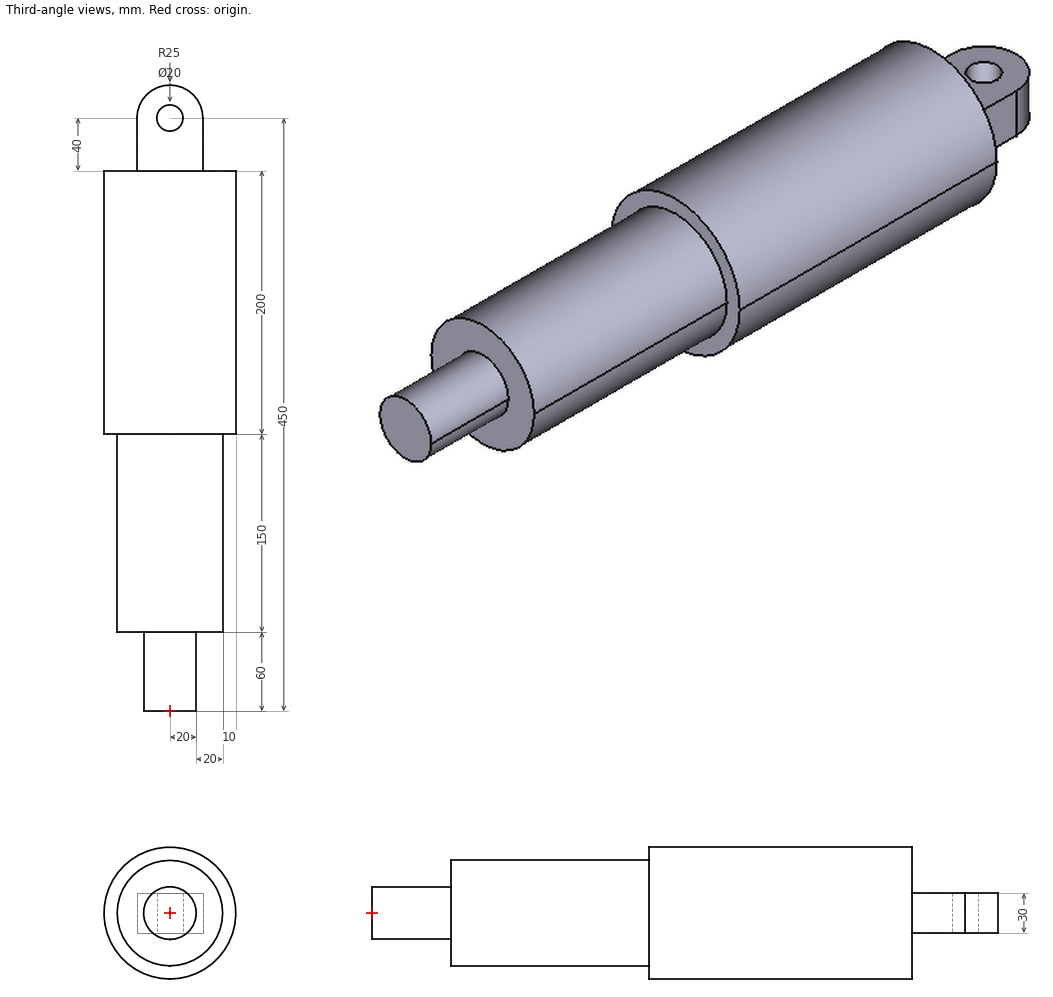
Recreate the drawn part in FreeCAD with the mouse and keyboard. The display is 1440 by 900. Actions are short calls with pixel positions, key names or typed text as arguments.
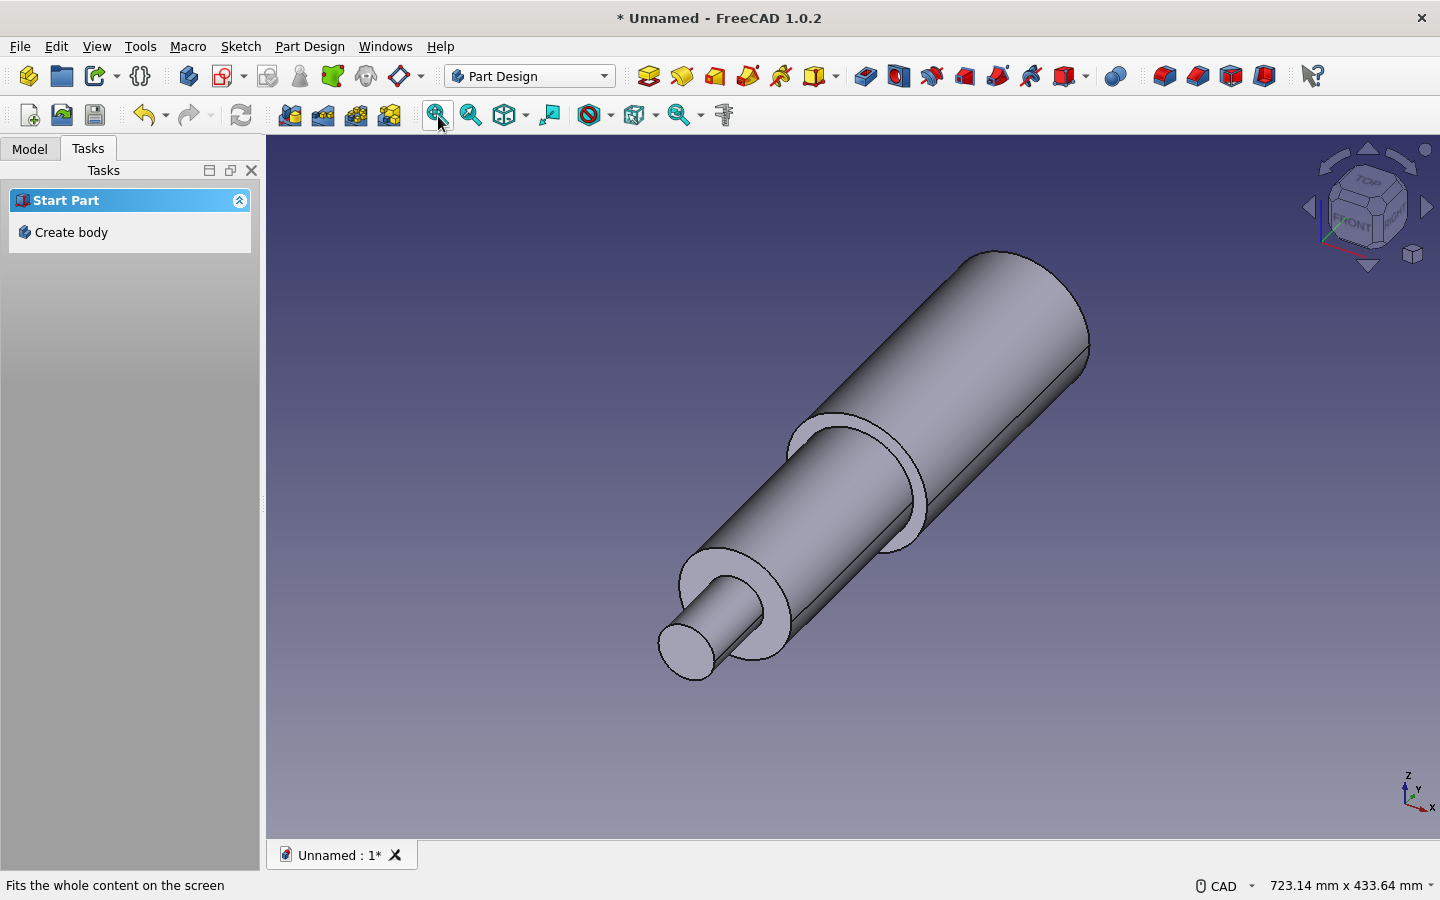
click(222, 76)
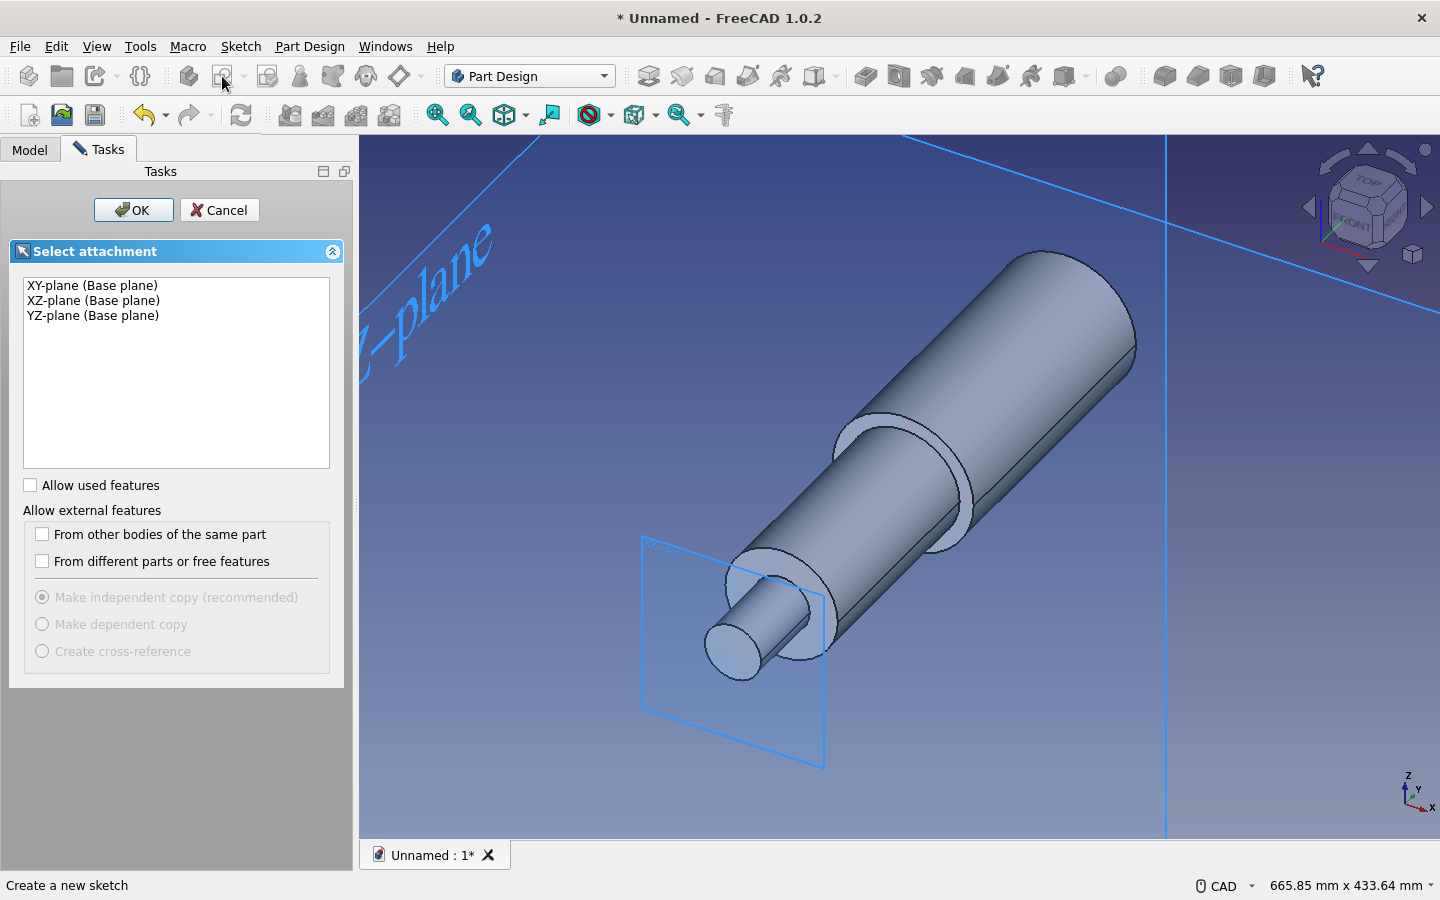
click(84, 286)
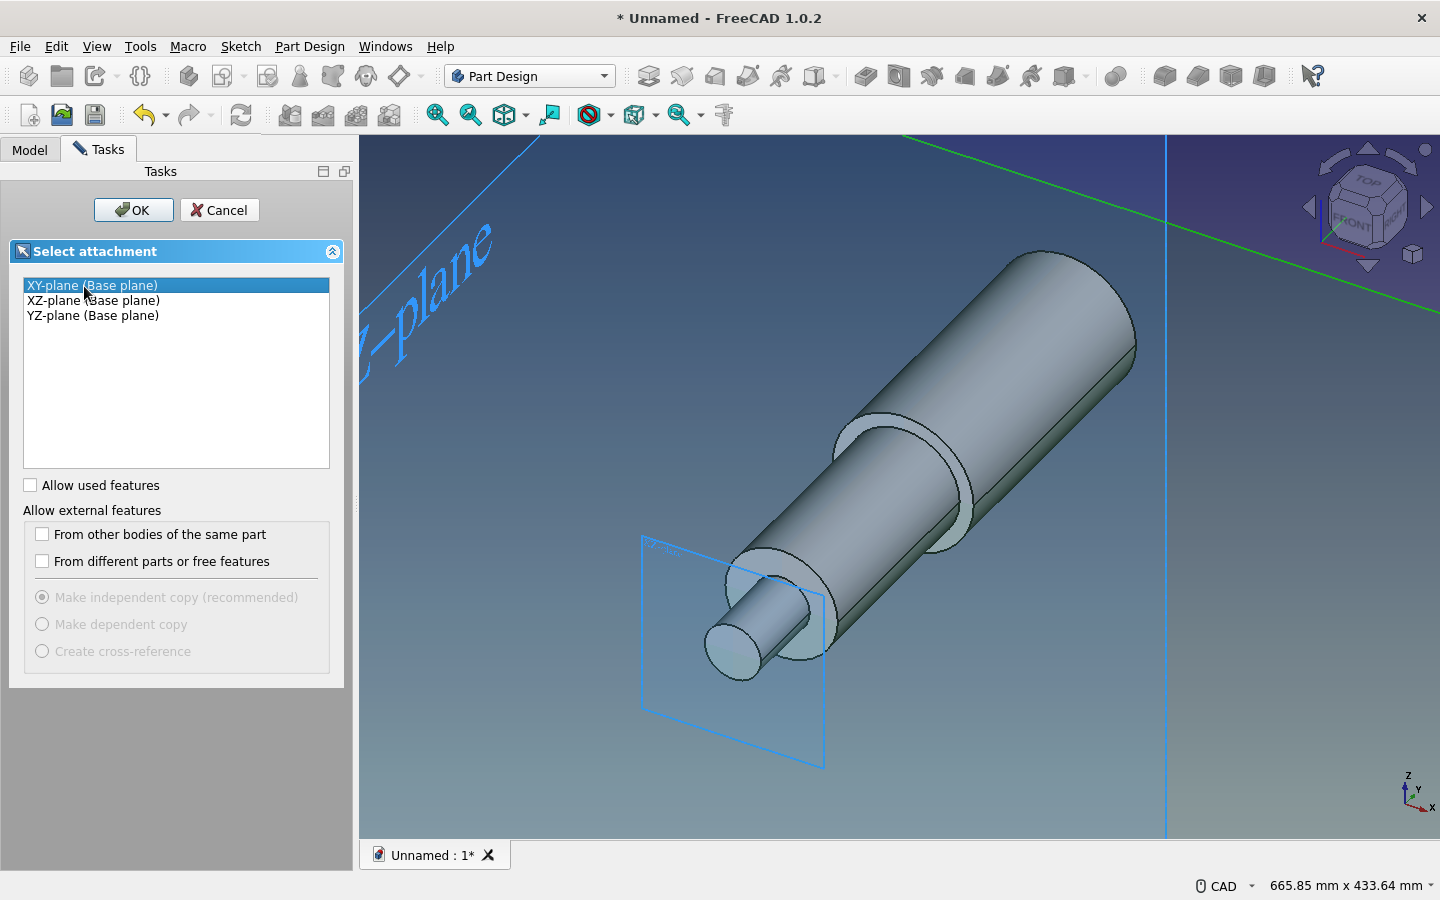
click(134, 210)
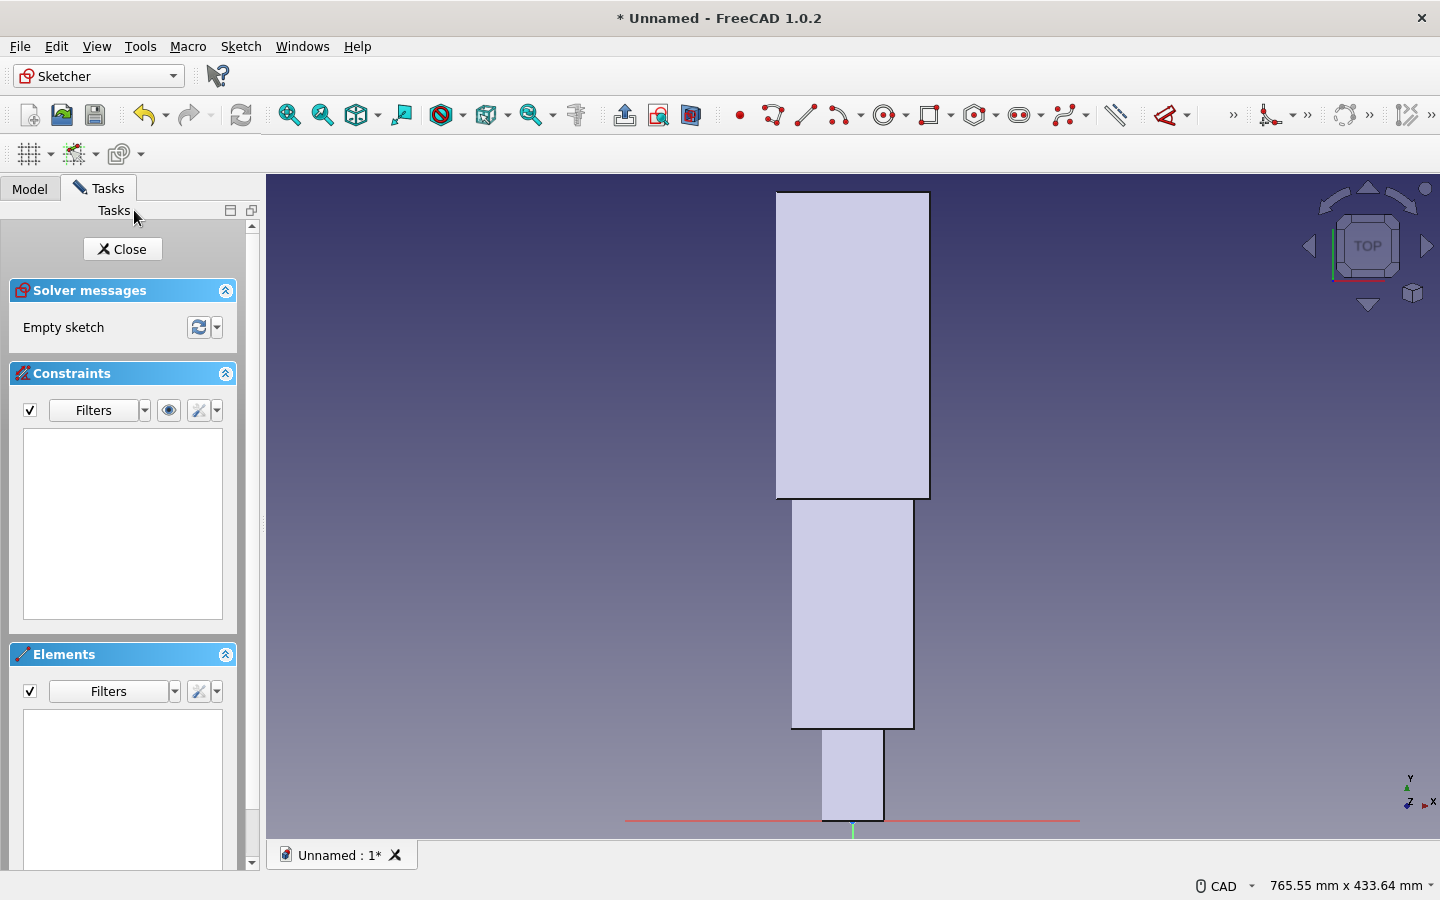
click(691, 116)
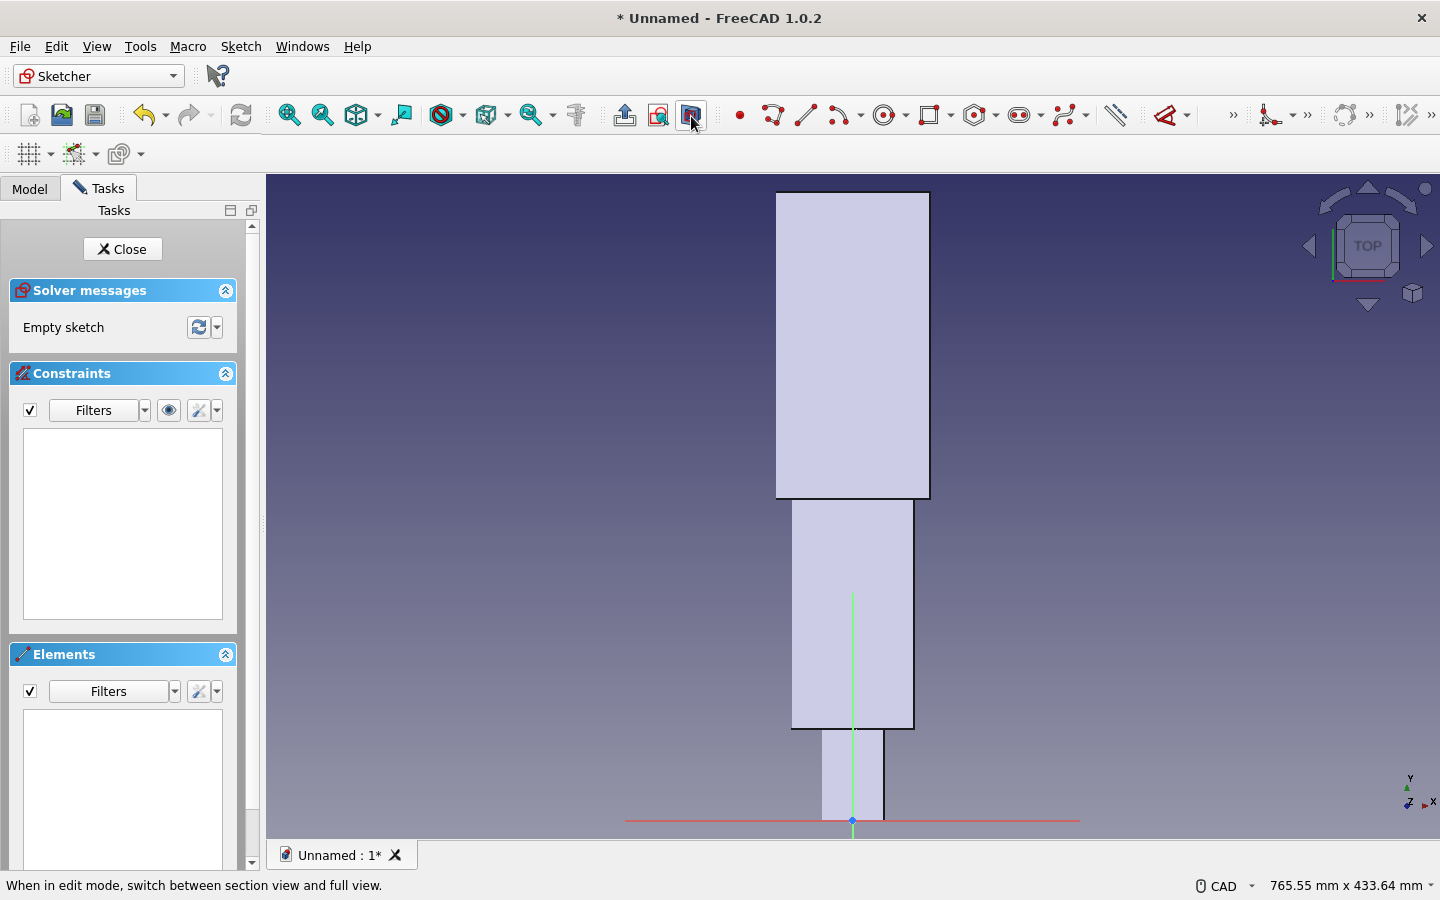
scroll(784, 506, down, 5)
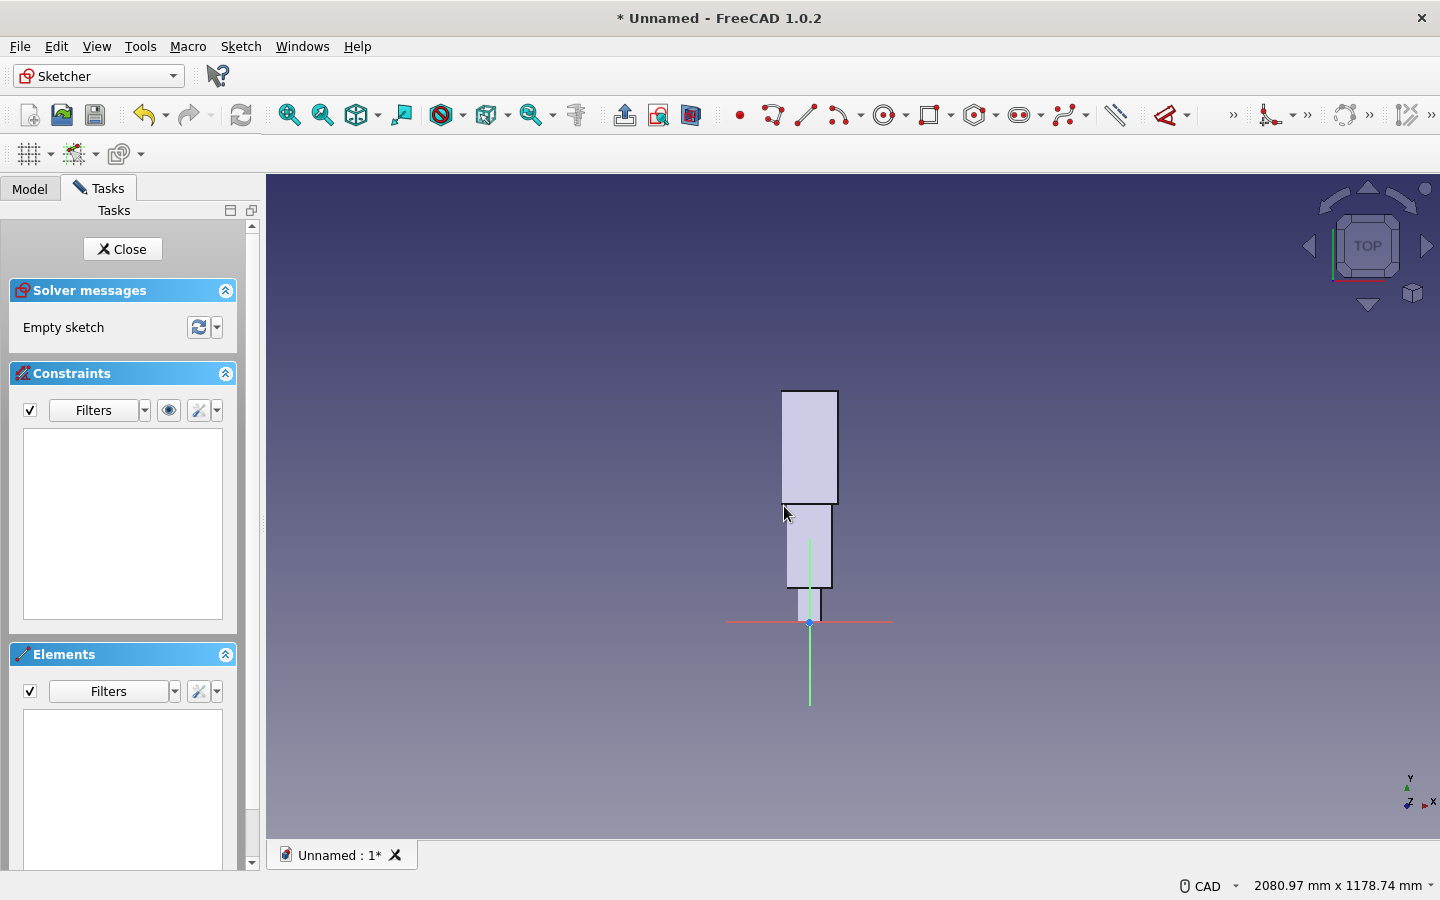
scroll(812, 359, up, 12)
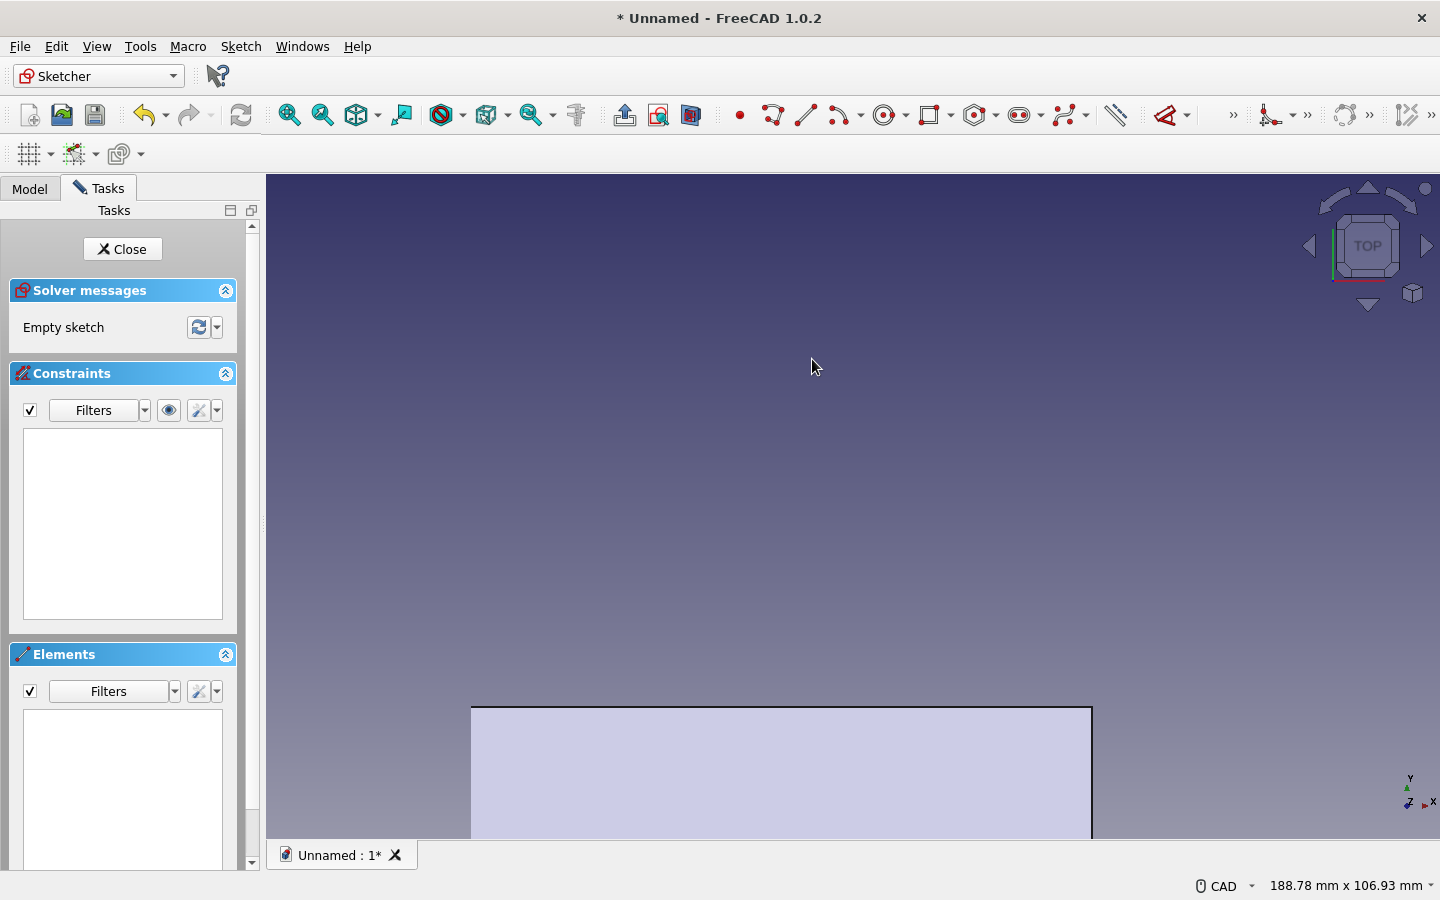
click(773, 116)